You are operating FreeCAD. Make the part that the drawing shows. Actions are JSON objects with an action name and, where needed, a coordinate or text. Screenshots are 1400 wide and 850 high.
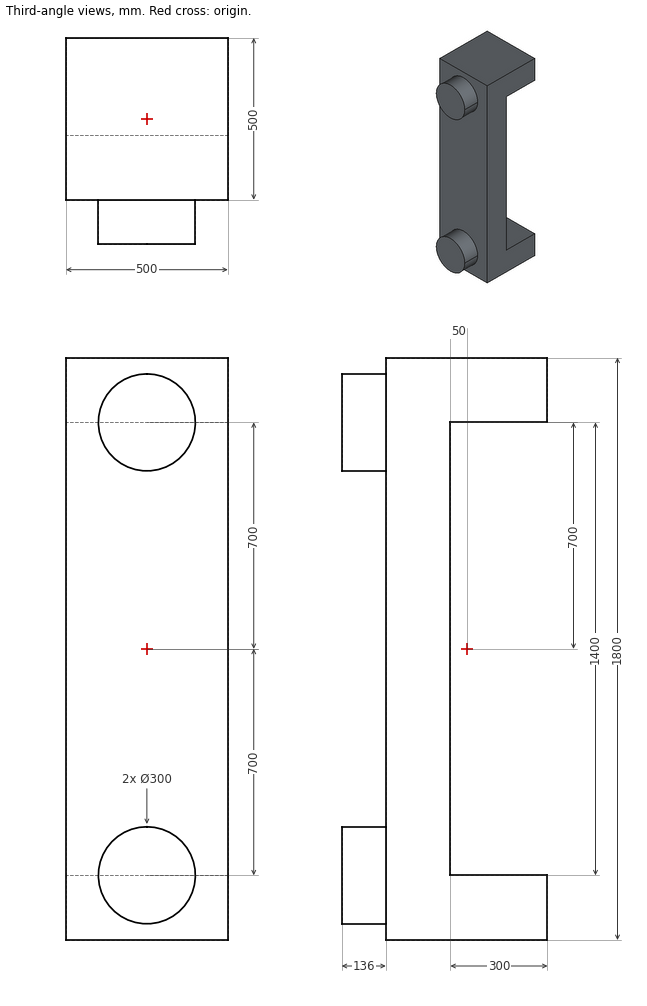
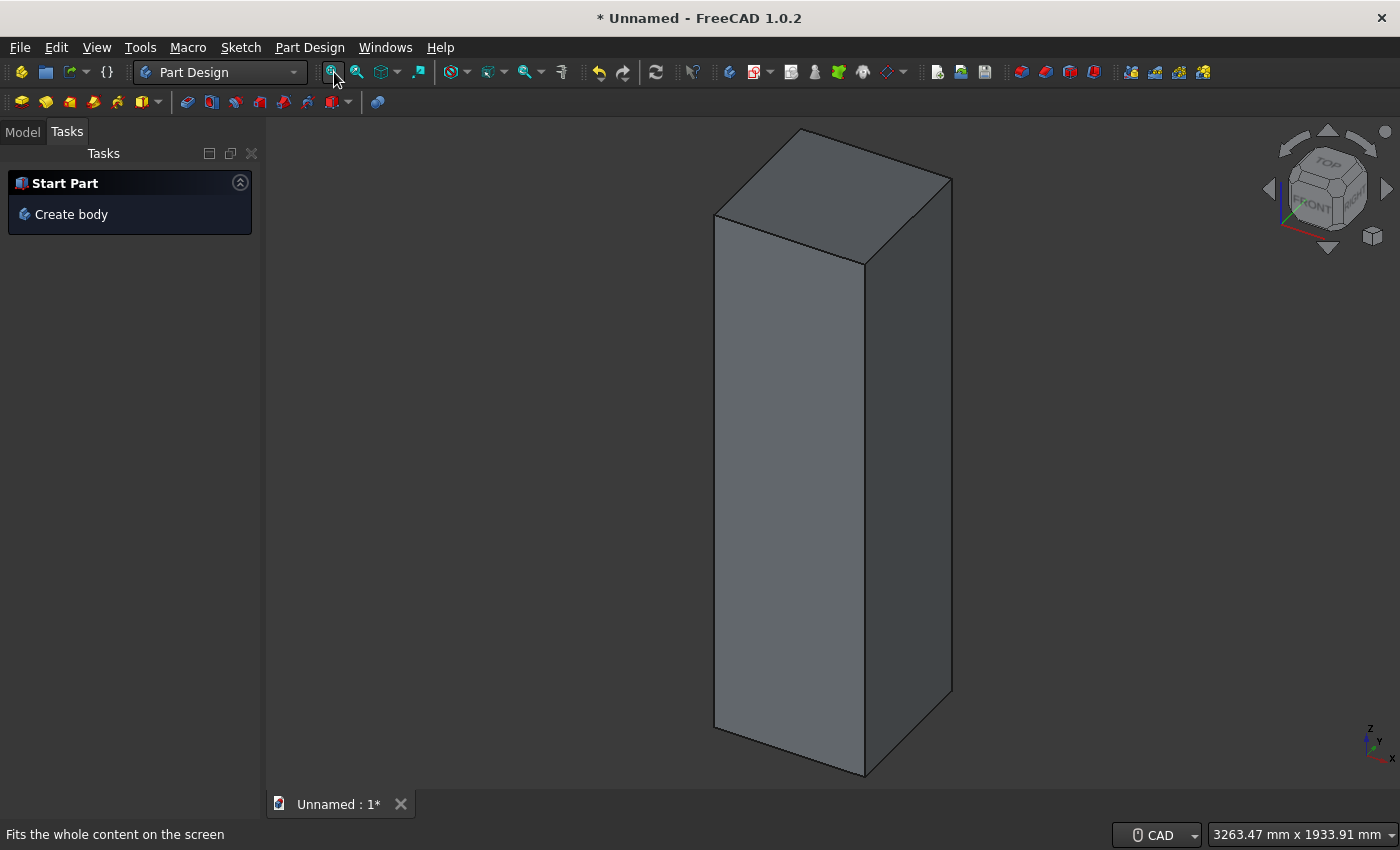
{"action": "left_click", "coordinate": [790, 349]}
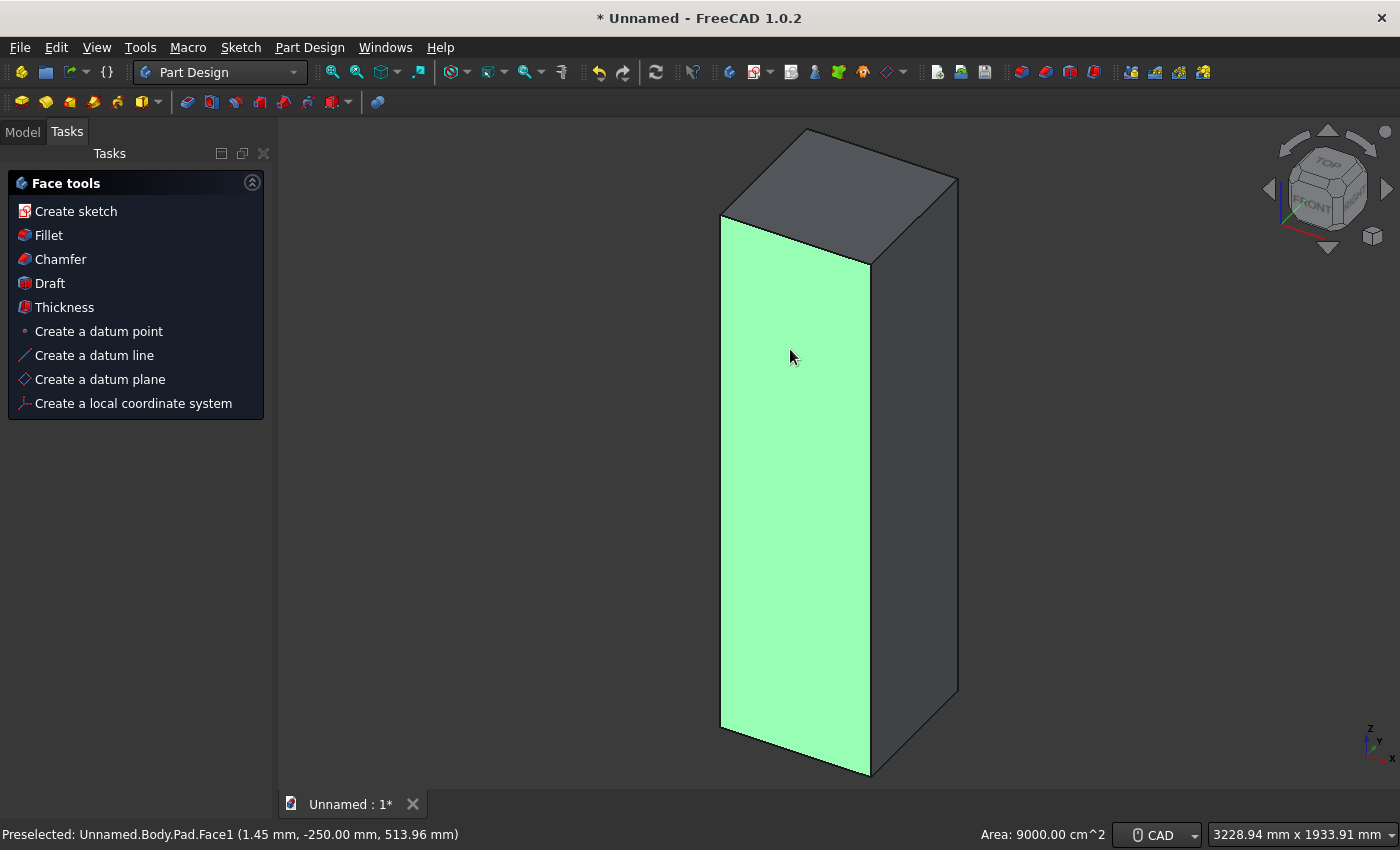
{"action": "left_click", "coordinate": [754, 72]}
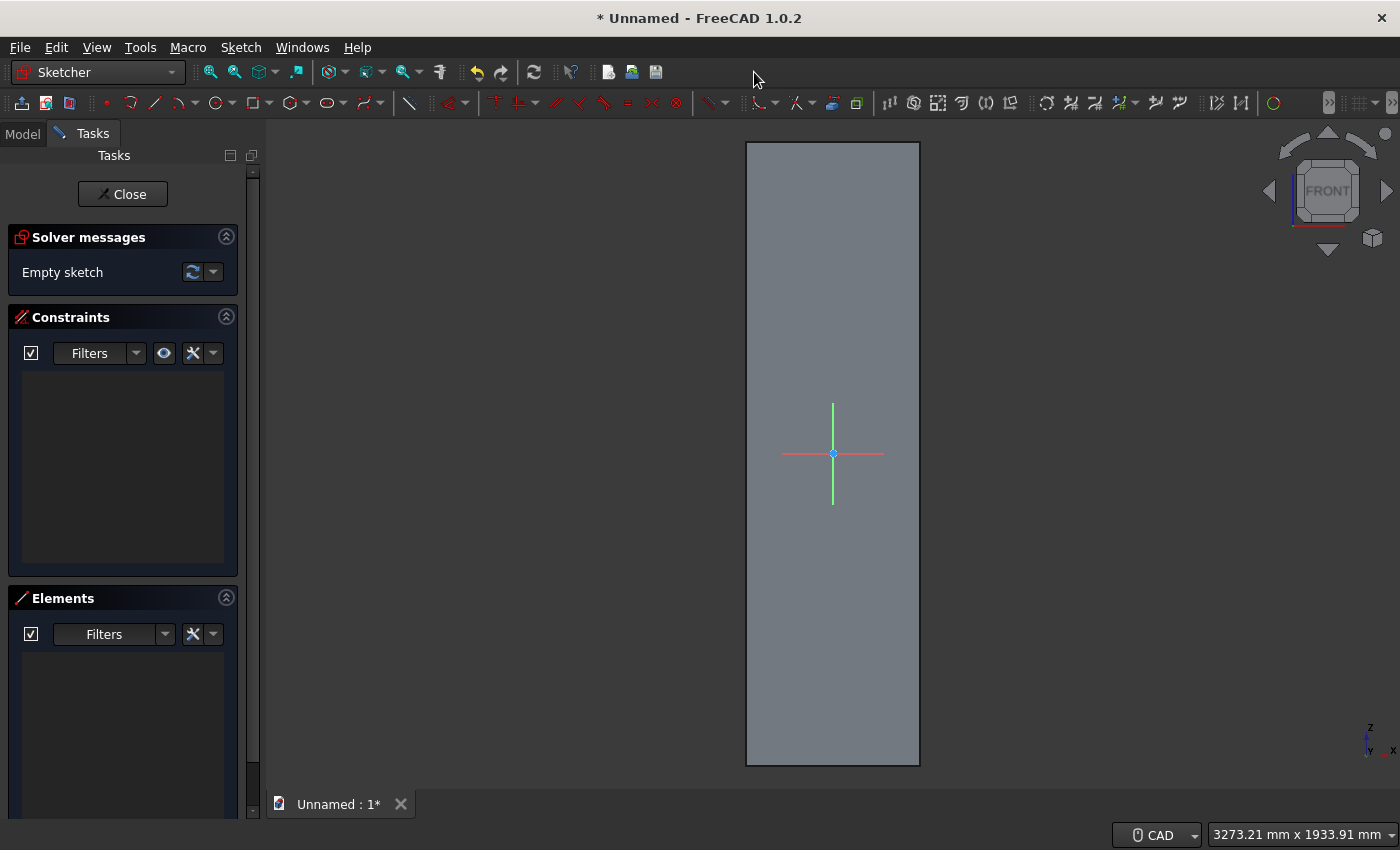
{"action": "scroll", "coordinate": [625, 454], "scroll_direction": "down", "scroll_amount": 2}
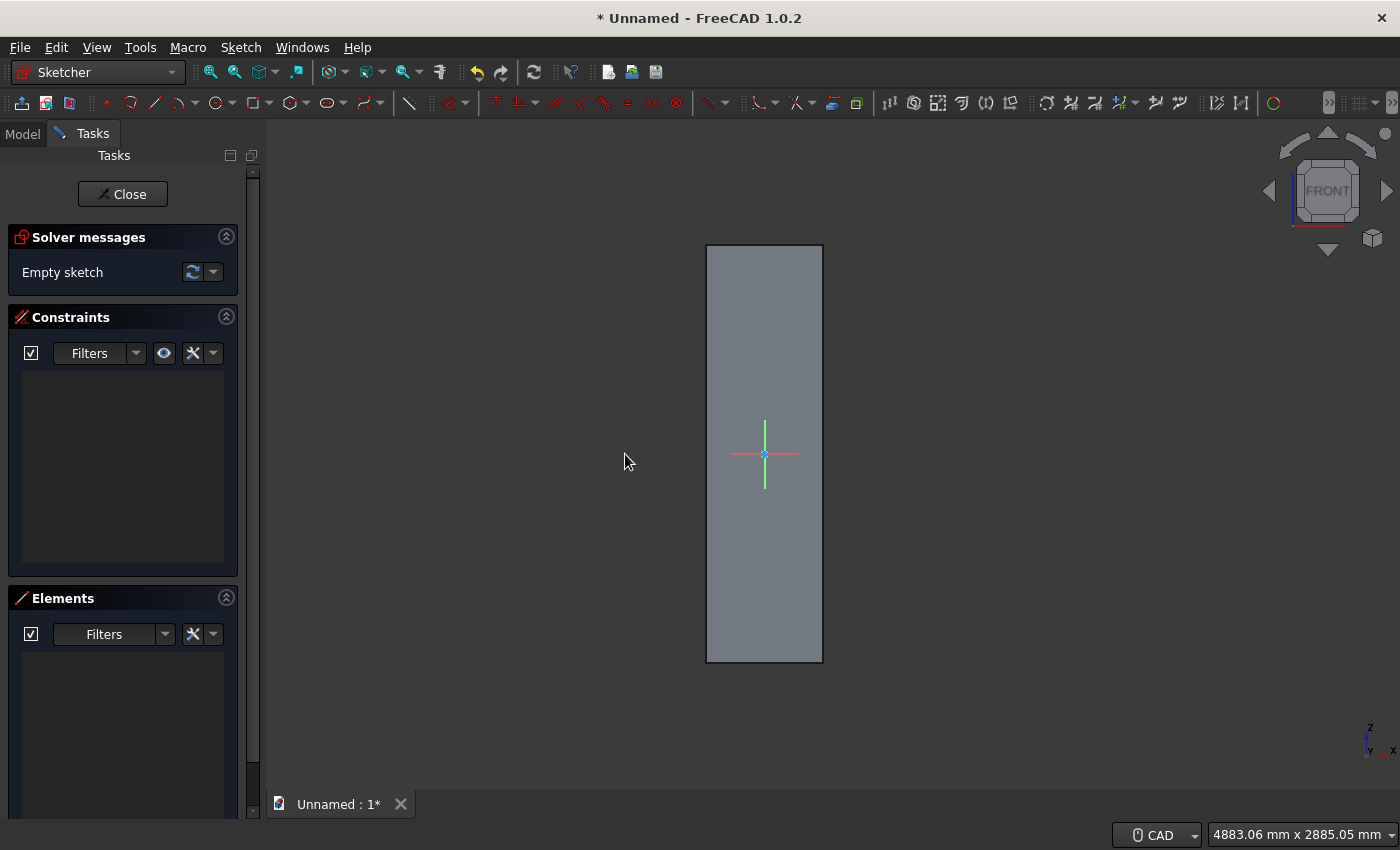
{"action": "left_click", "coordinate": [216, 104]}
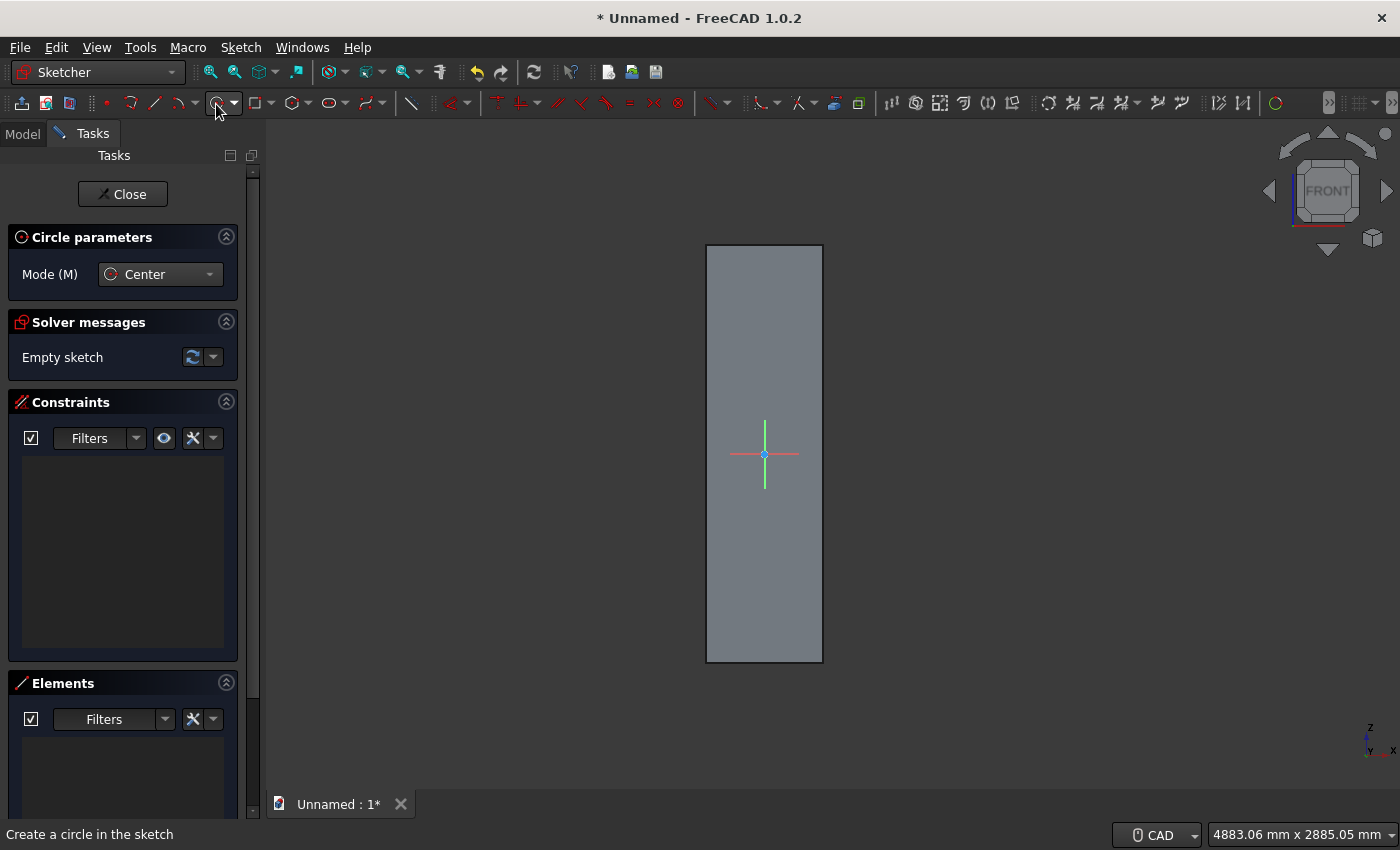
{"action": "left_click", "coordinate": [765, 617]}
{"action": "left_click", "coordinate": [789, 592]}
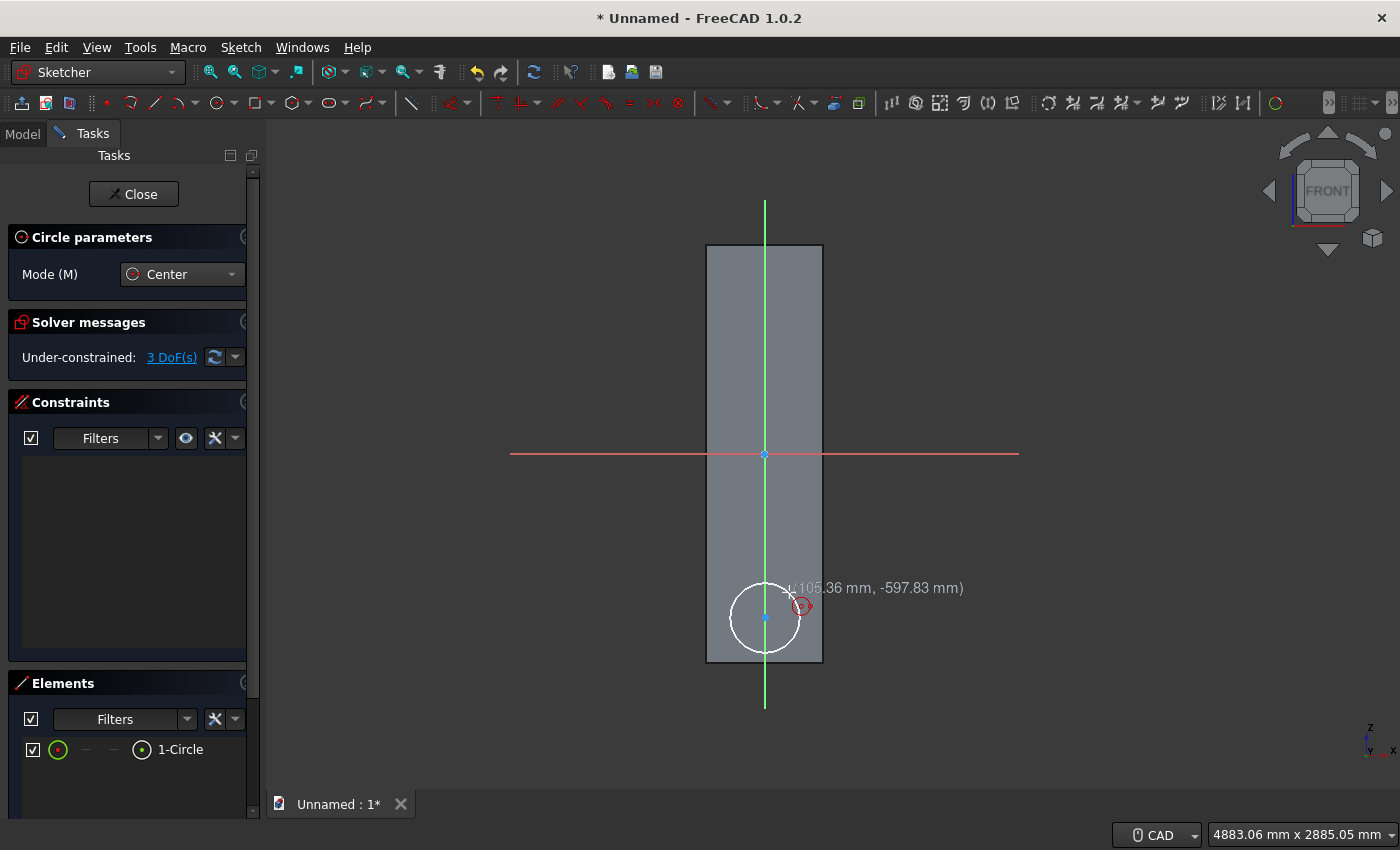
{"action": "left_click", "coordinate": [765, 292]}
{"action": "left_click", "coordinate": [789, 267]}
{"action": "key", "text": "Escape"}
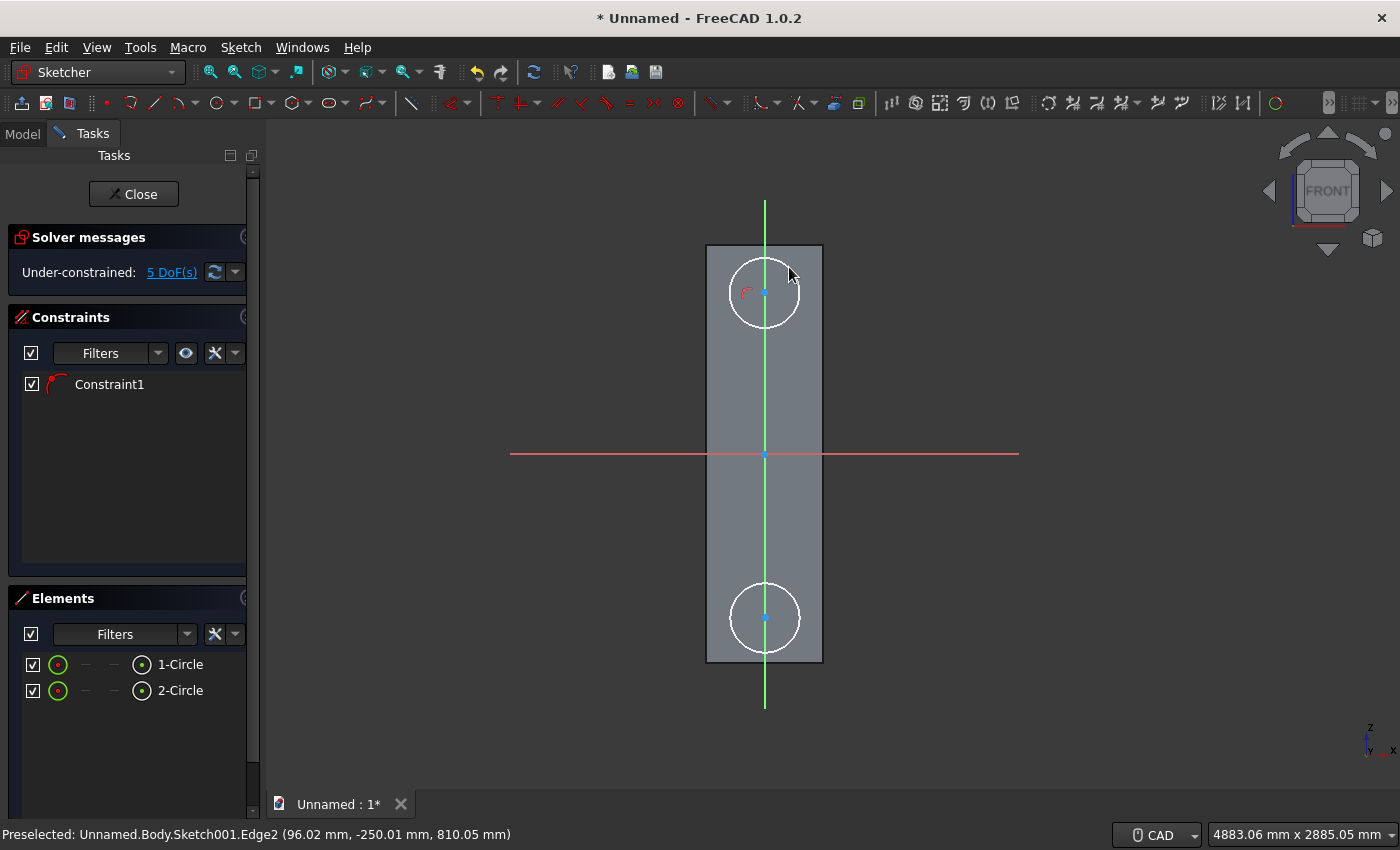
{"action": "left_click", "coordinate": [789, 593]}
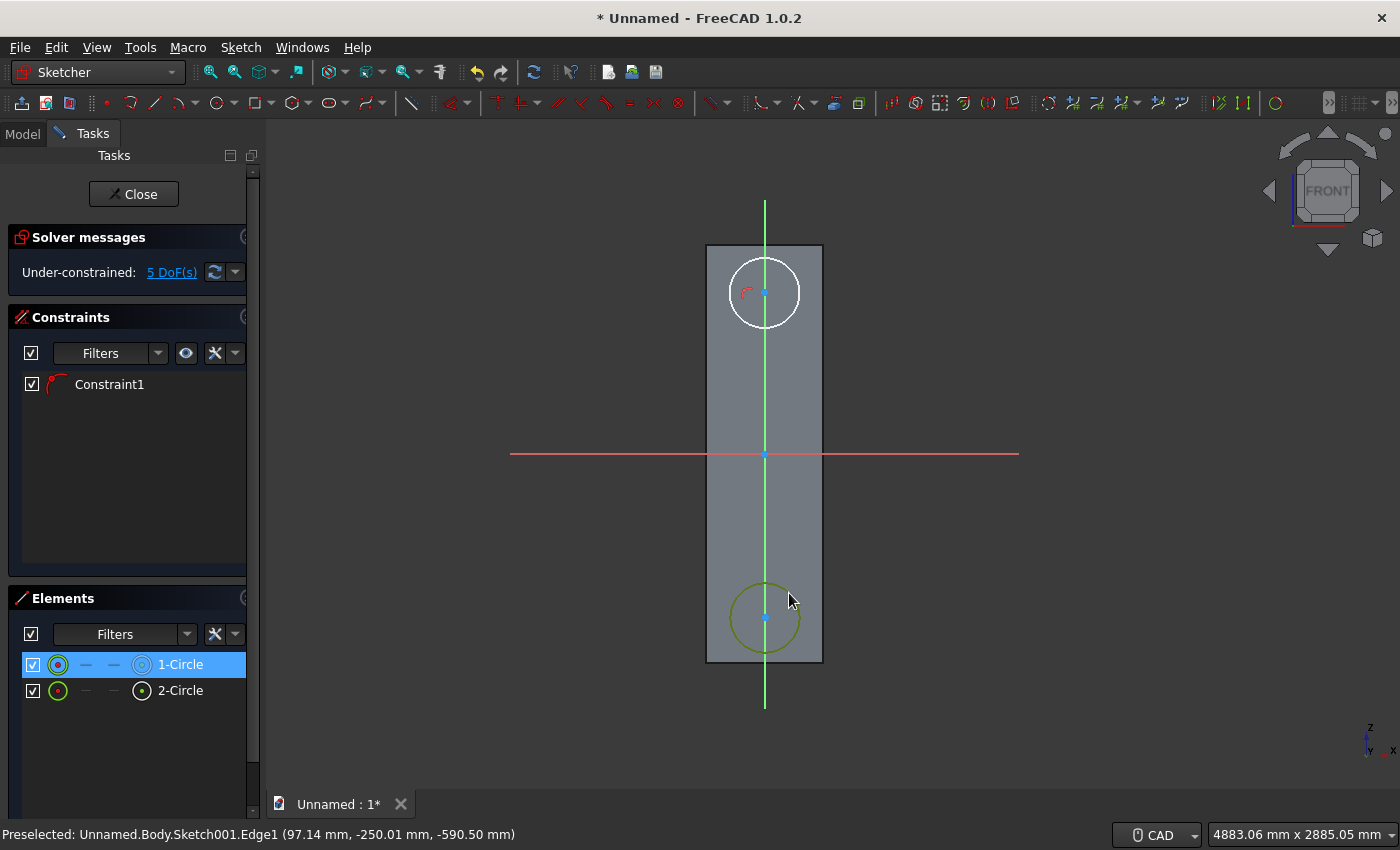
{"action": "left_click", "coordinate": [789, 268]}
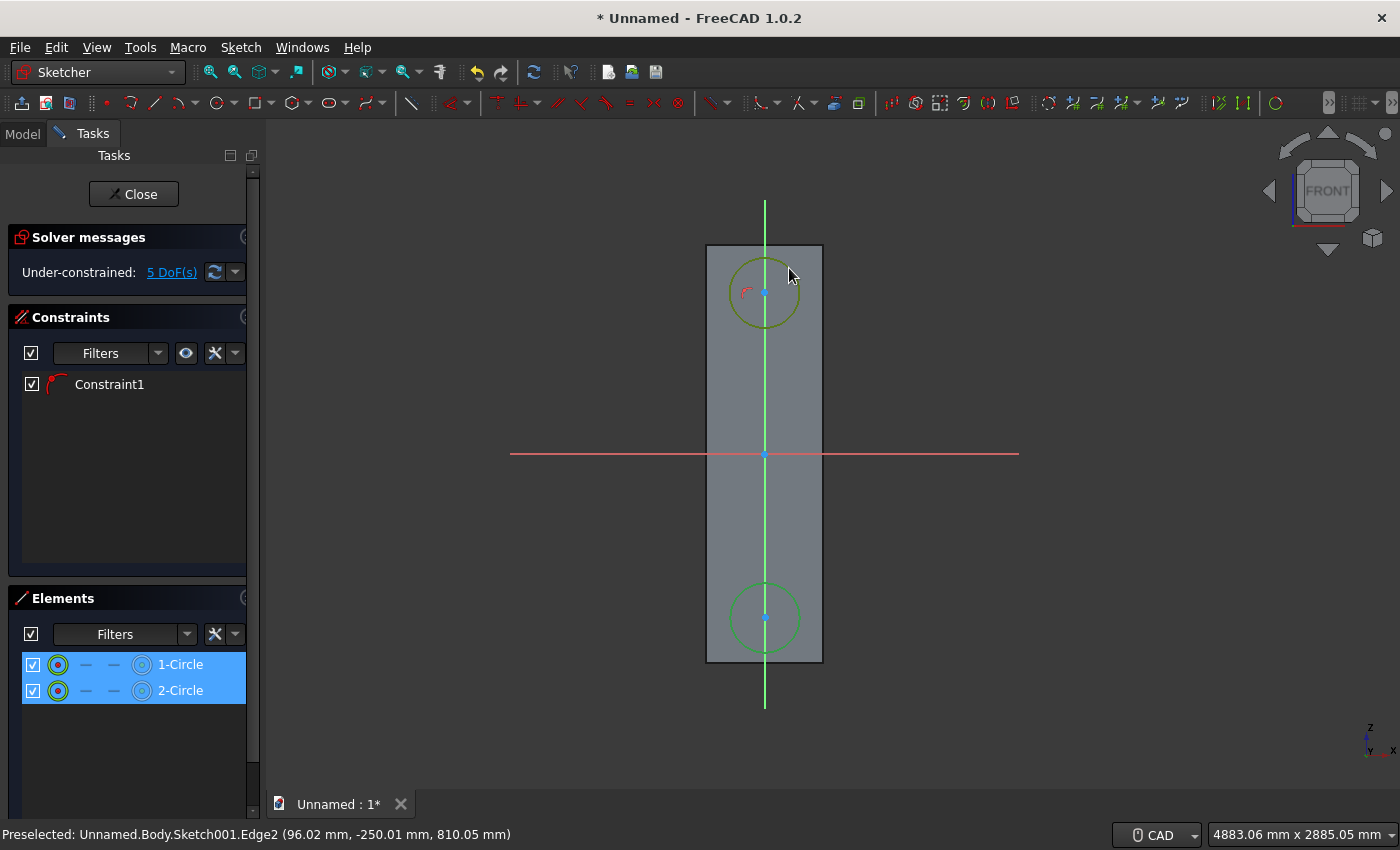
{"action": "left_click", "coordinate": [630, 104]}